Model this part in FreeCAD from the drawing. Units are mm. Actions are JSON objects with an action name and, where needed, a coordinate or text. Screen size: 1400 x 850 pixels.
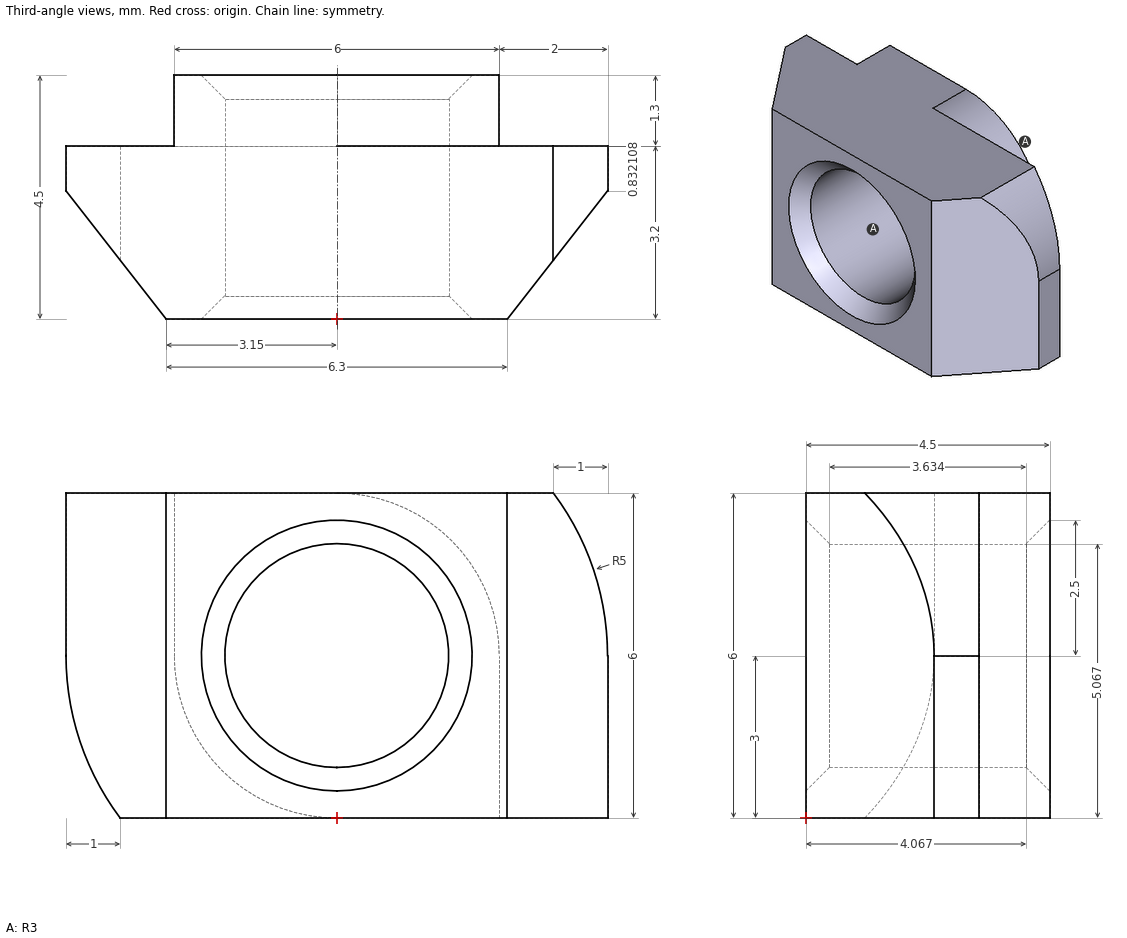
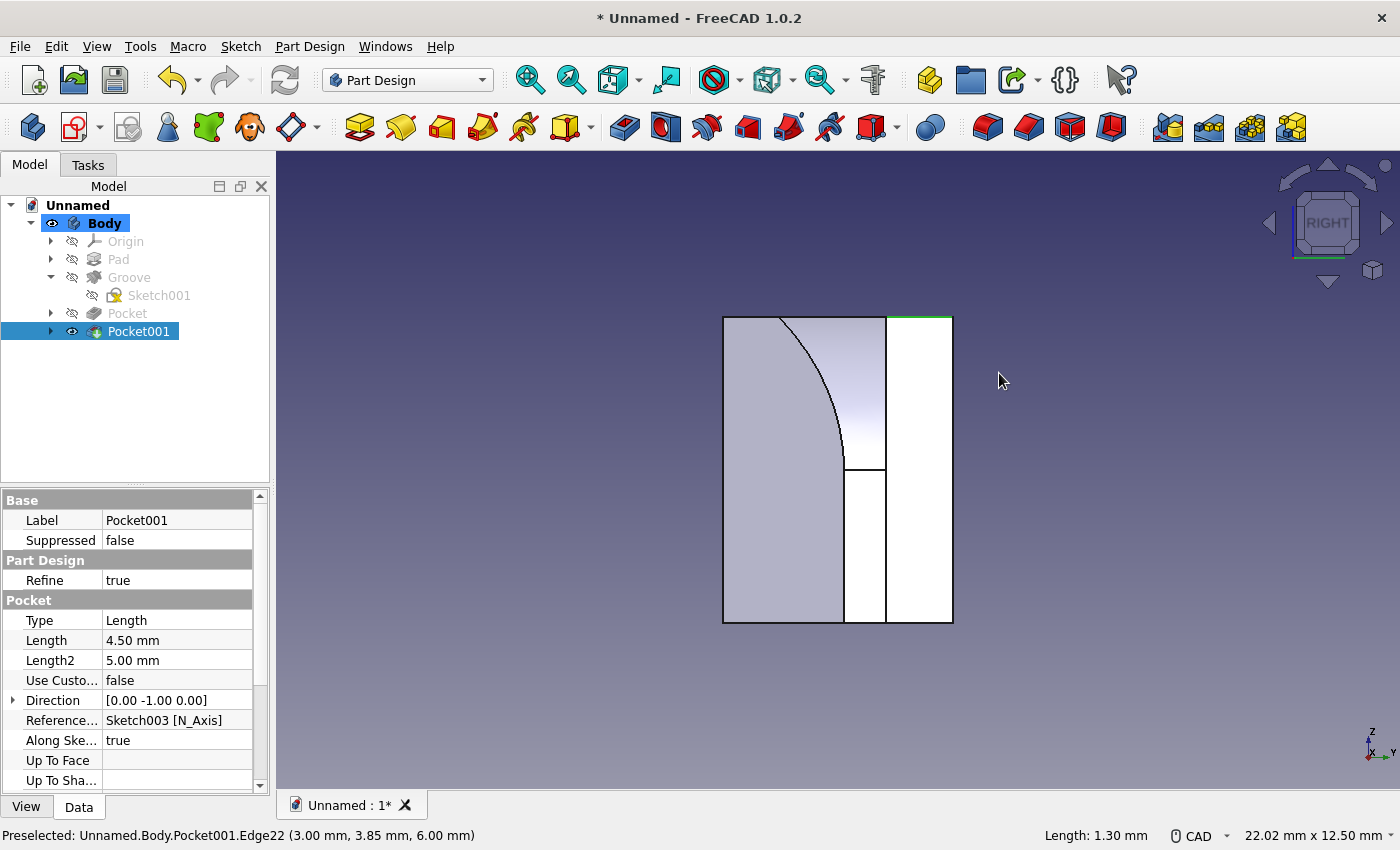
{"action": "key", "text": "5"}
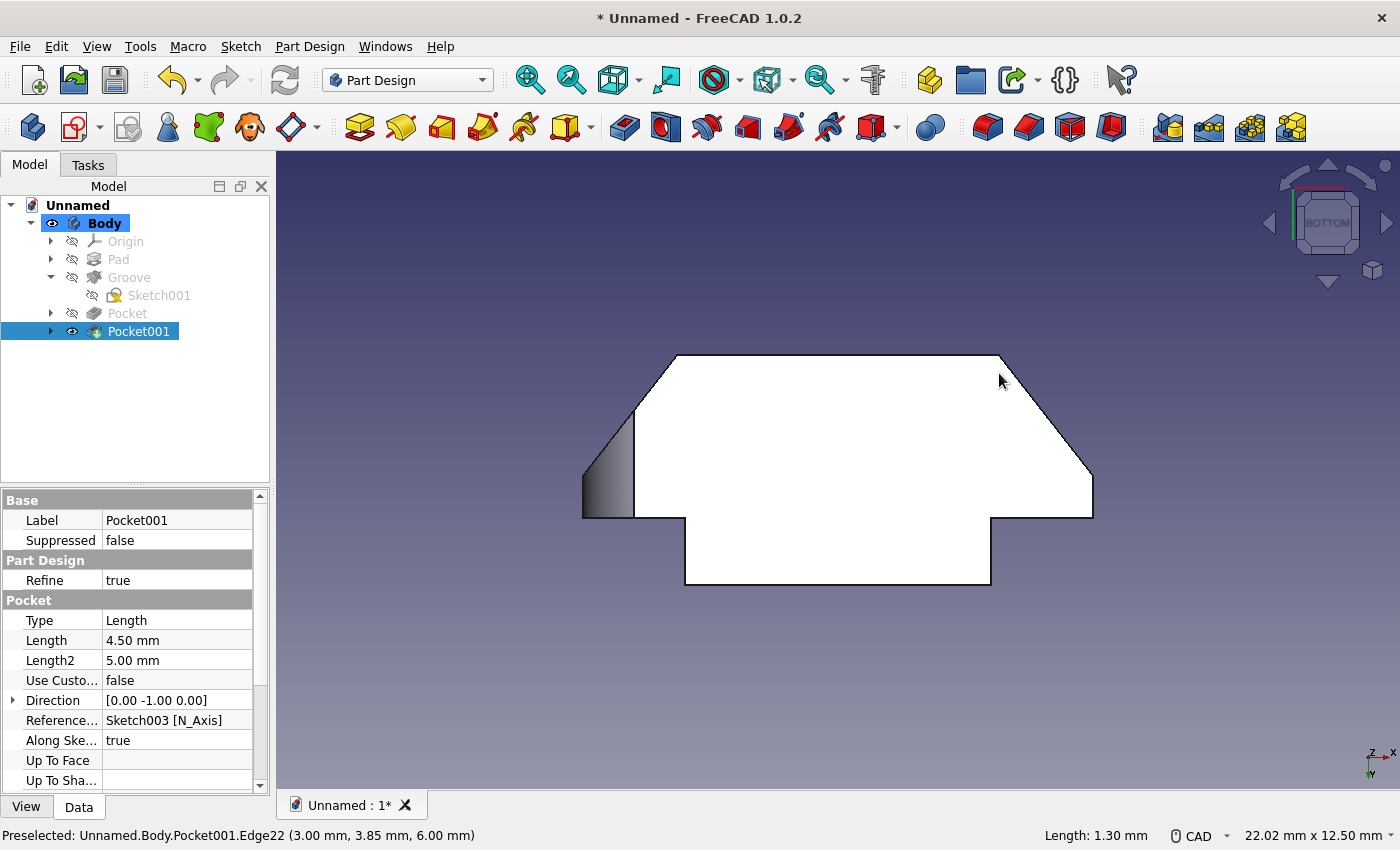
{"action": "key", "text": "4"}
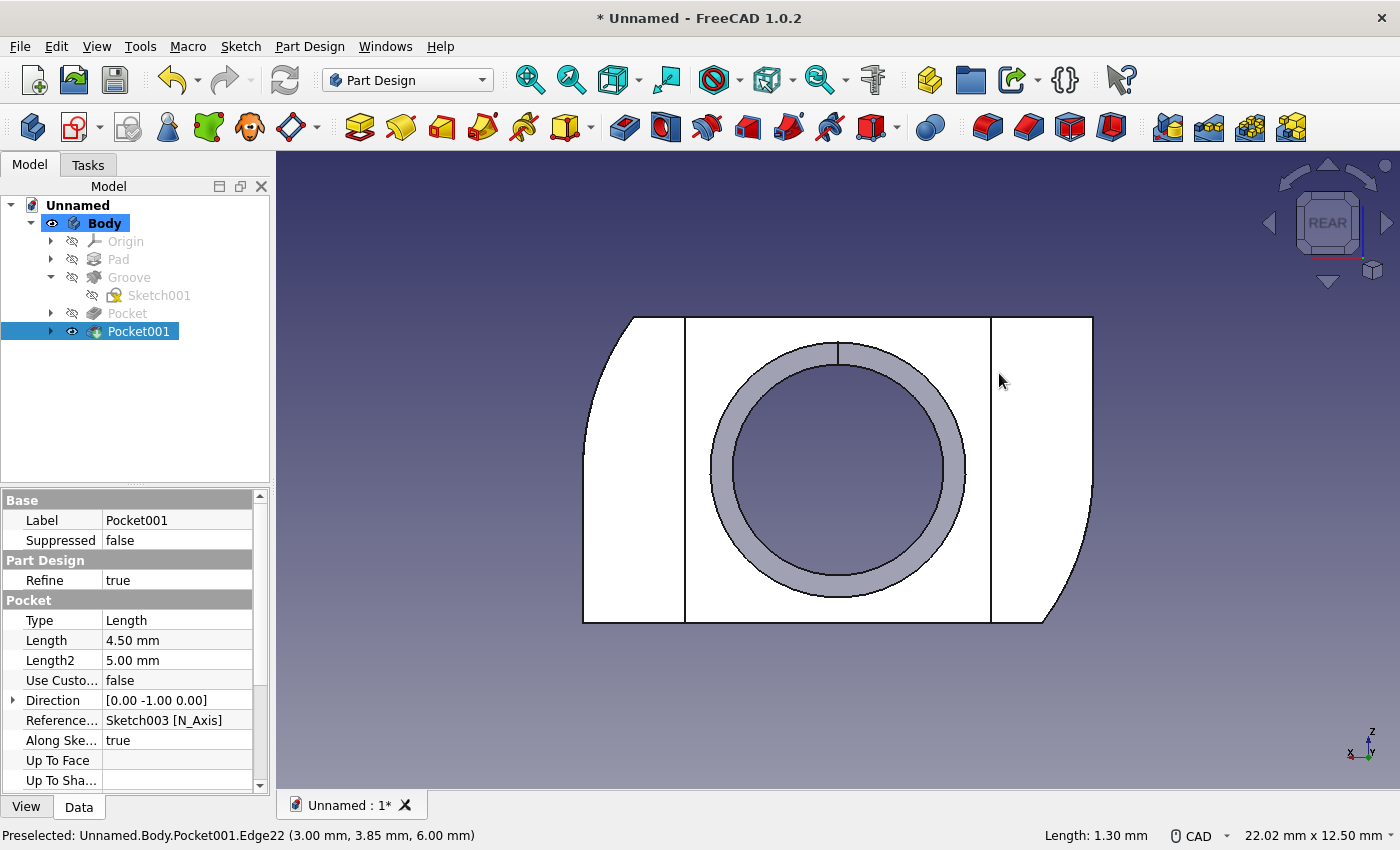
{"action": "key", "text": "6"}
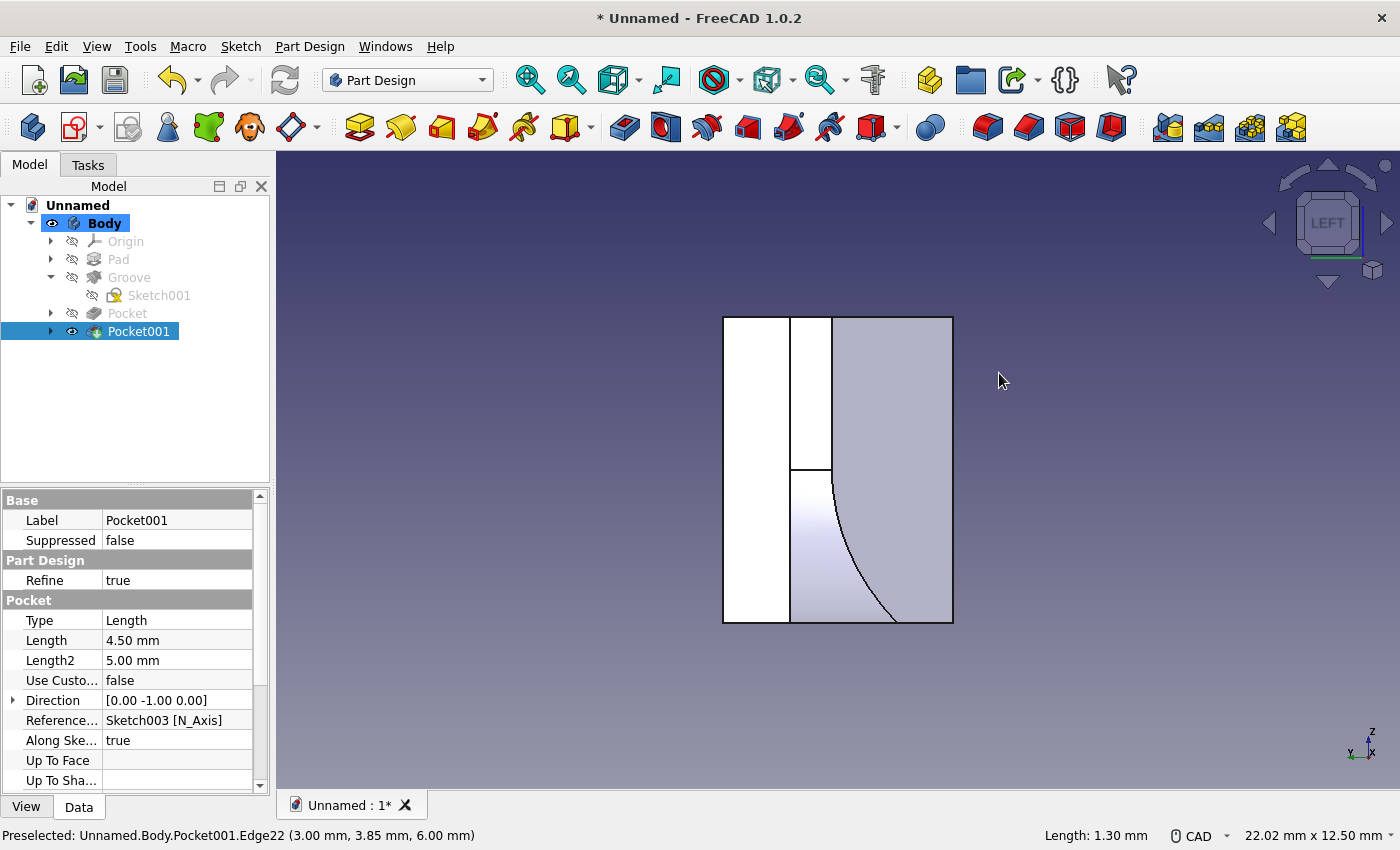
{"action": "left_click", "coordinate": [756, 622], "text": "ctrl"}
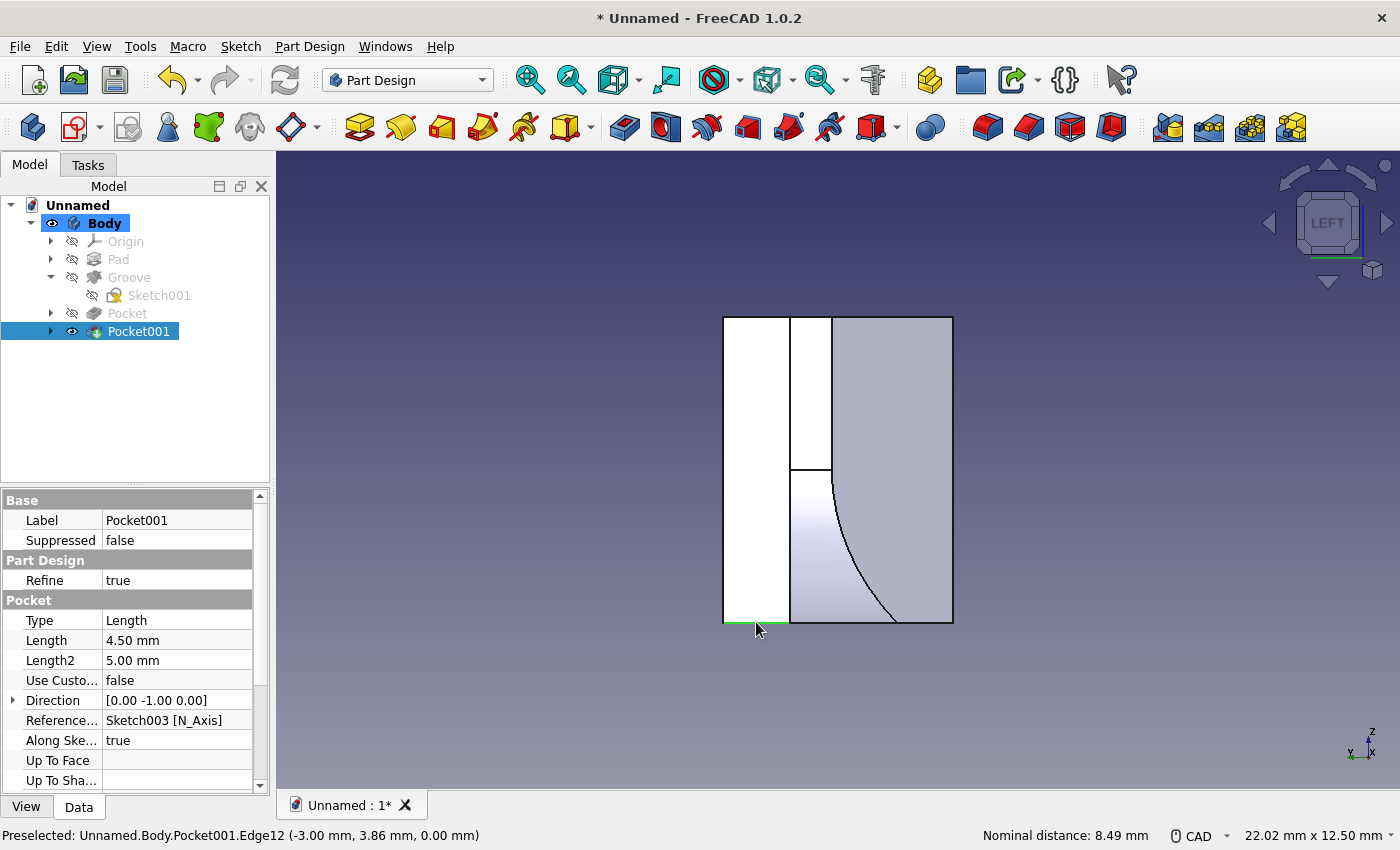
{"action": "left_click", "coordinate": [988, 128]}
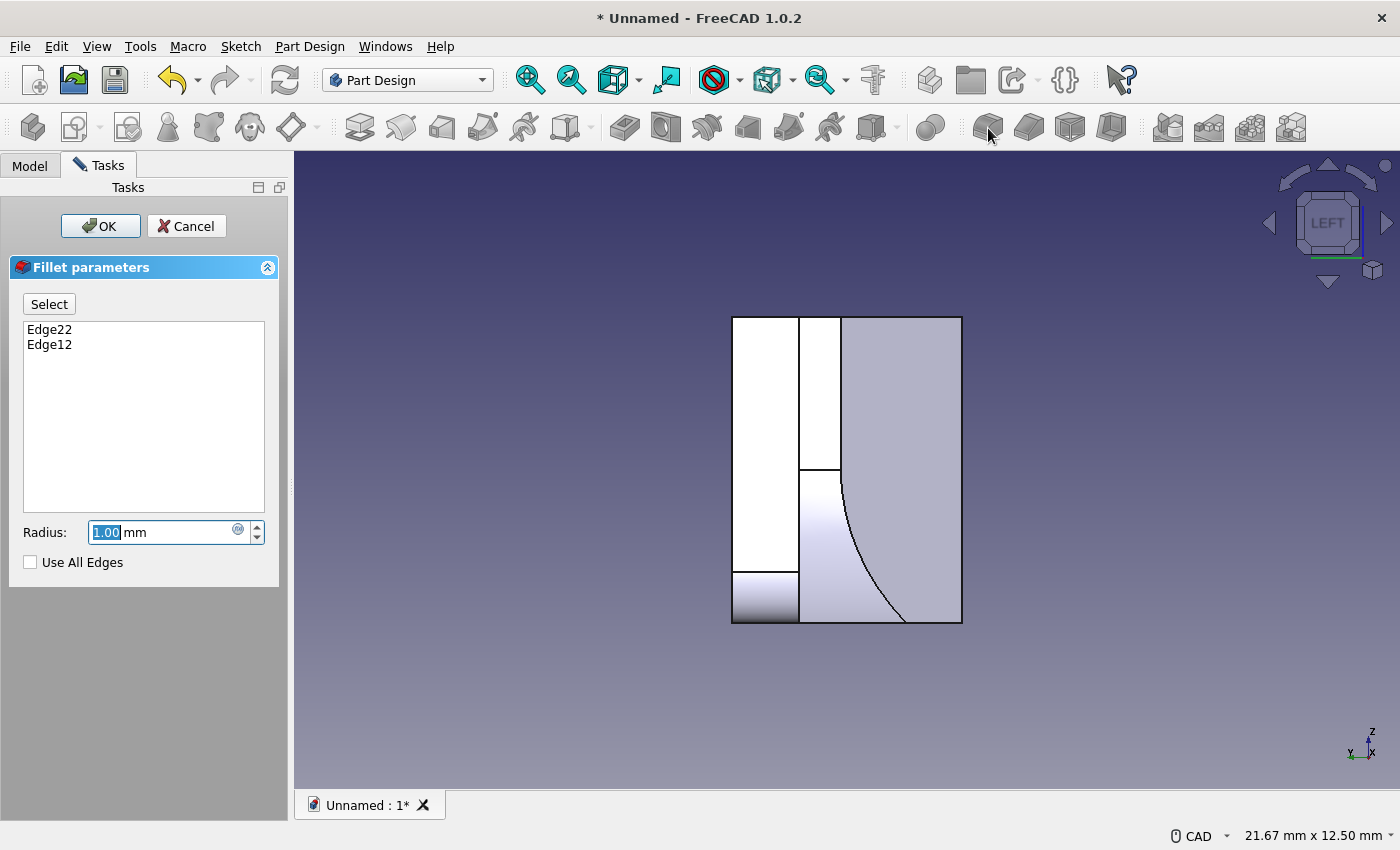
{"action": "type", "text": "3"}
{"action": "key", "text": "Tab"}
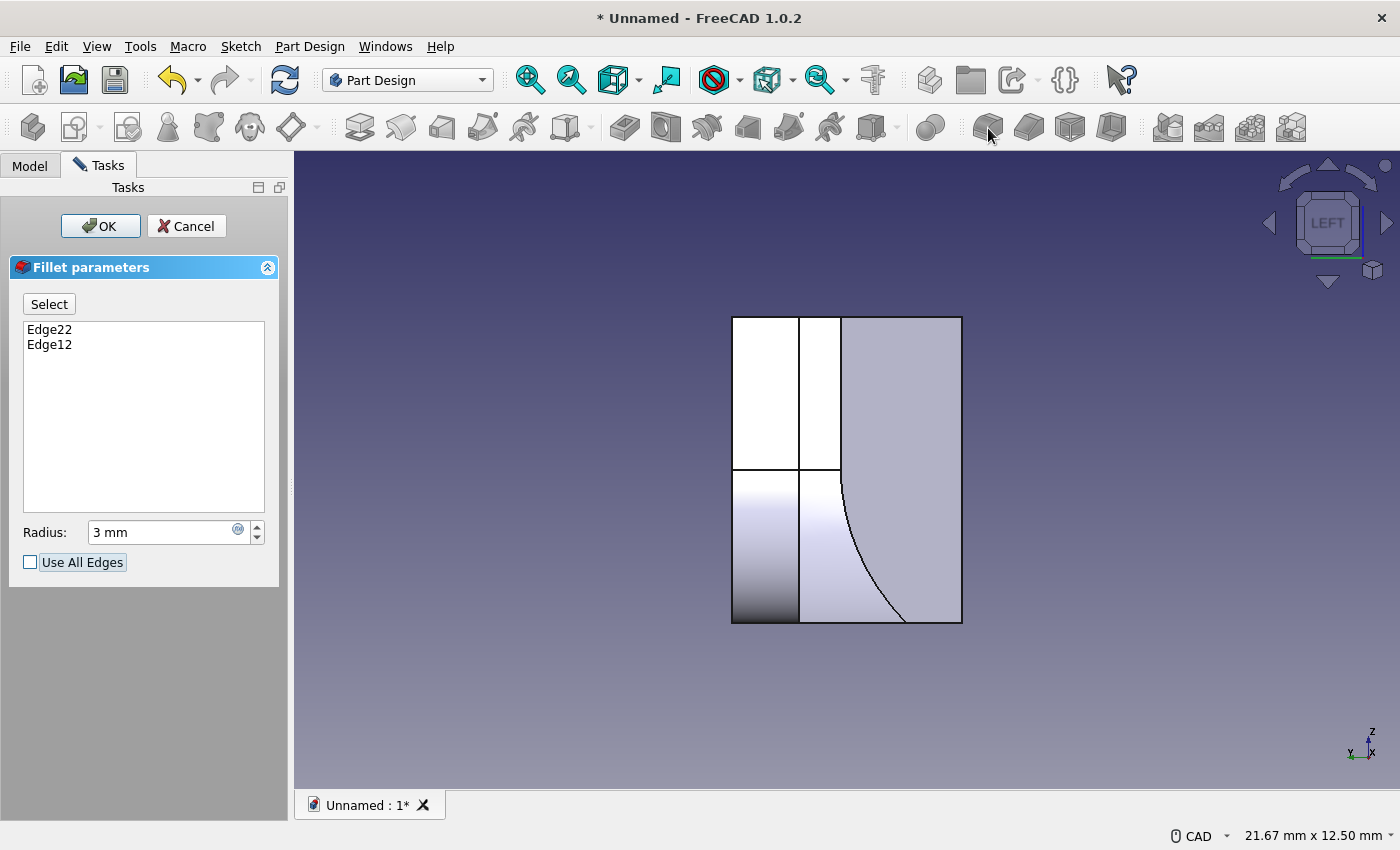
{"action": "left_click", "coordinate": [101, 226]}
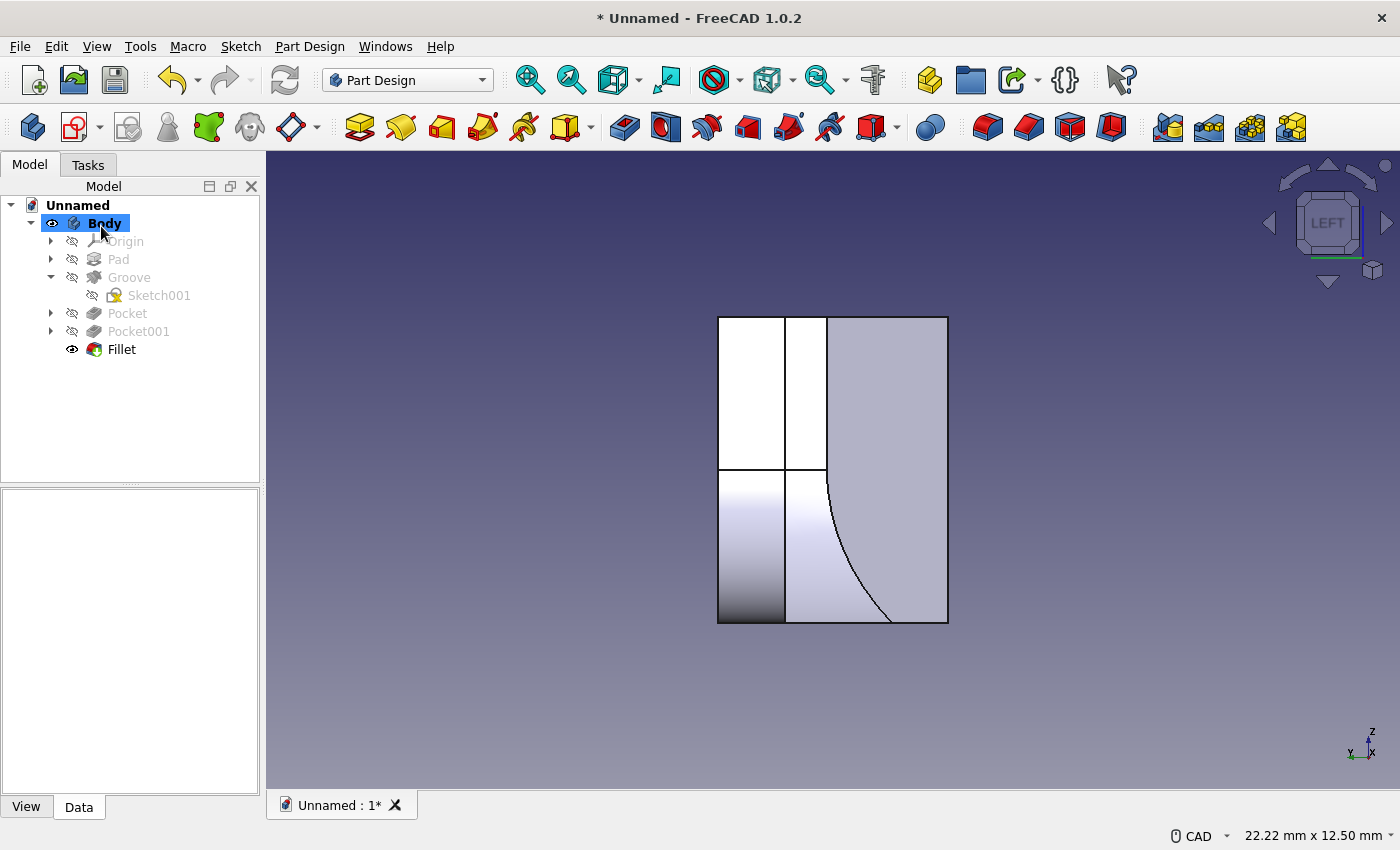
{"action": "key", "text": "0"}